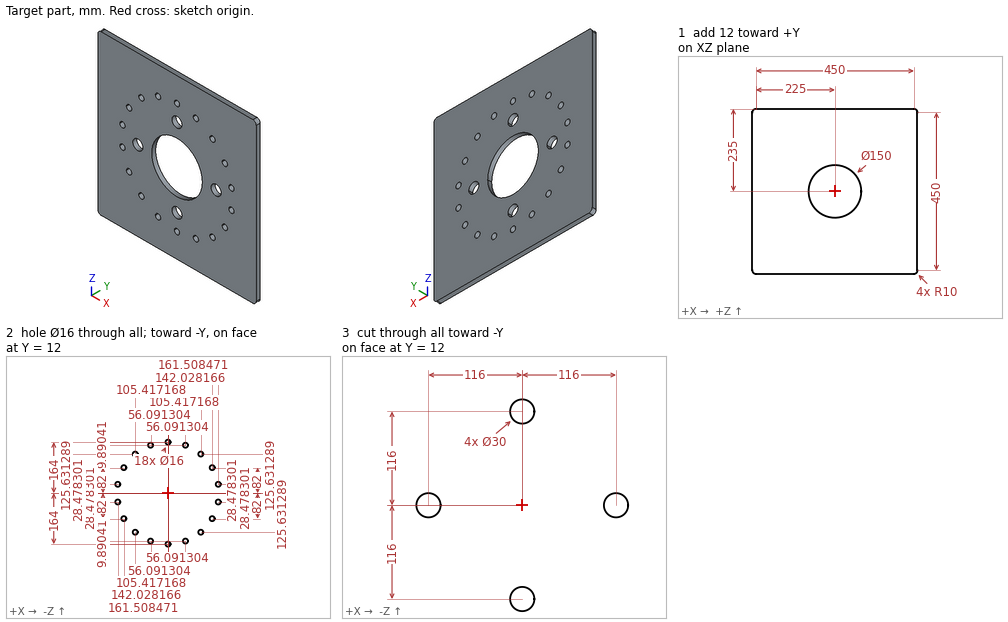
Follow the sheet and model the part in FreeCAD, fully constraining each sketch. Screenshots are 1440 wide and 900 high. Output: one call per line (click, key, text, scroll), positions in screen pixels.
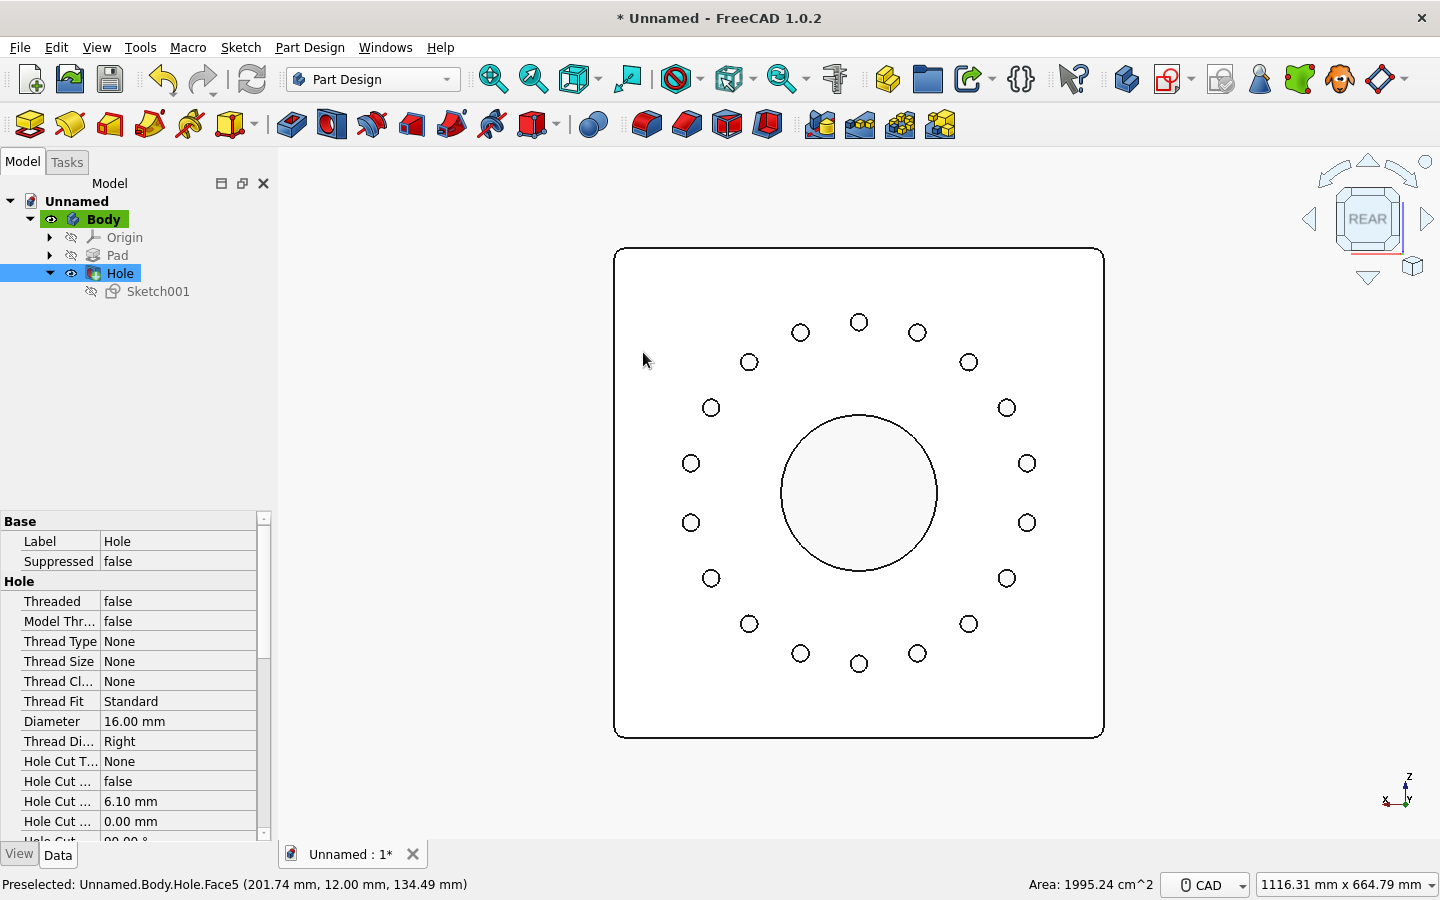
click(1168, 80)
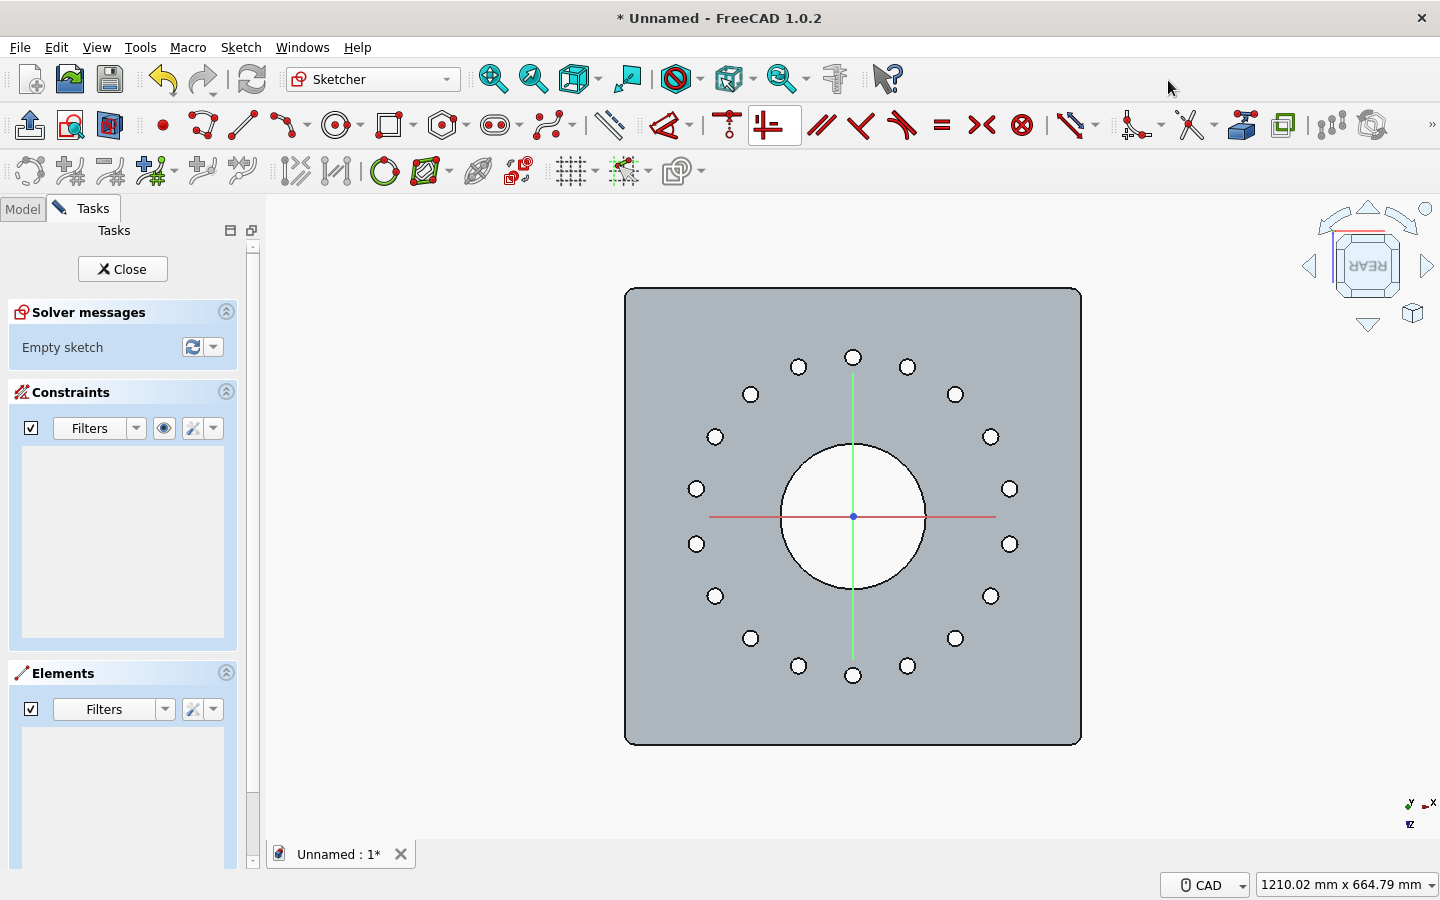
scroll(992, 516, up, 2)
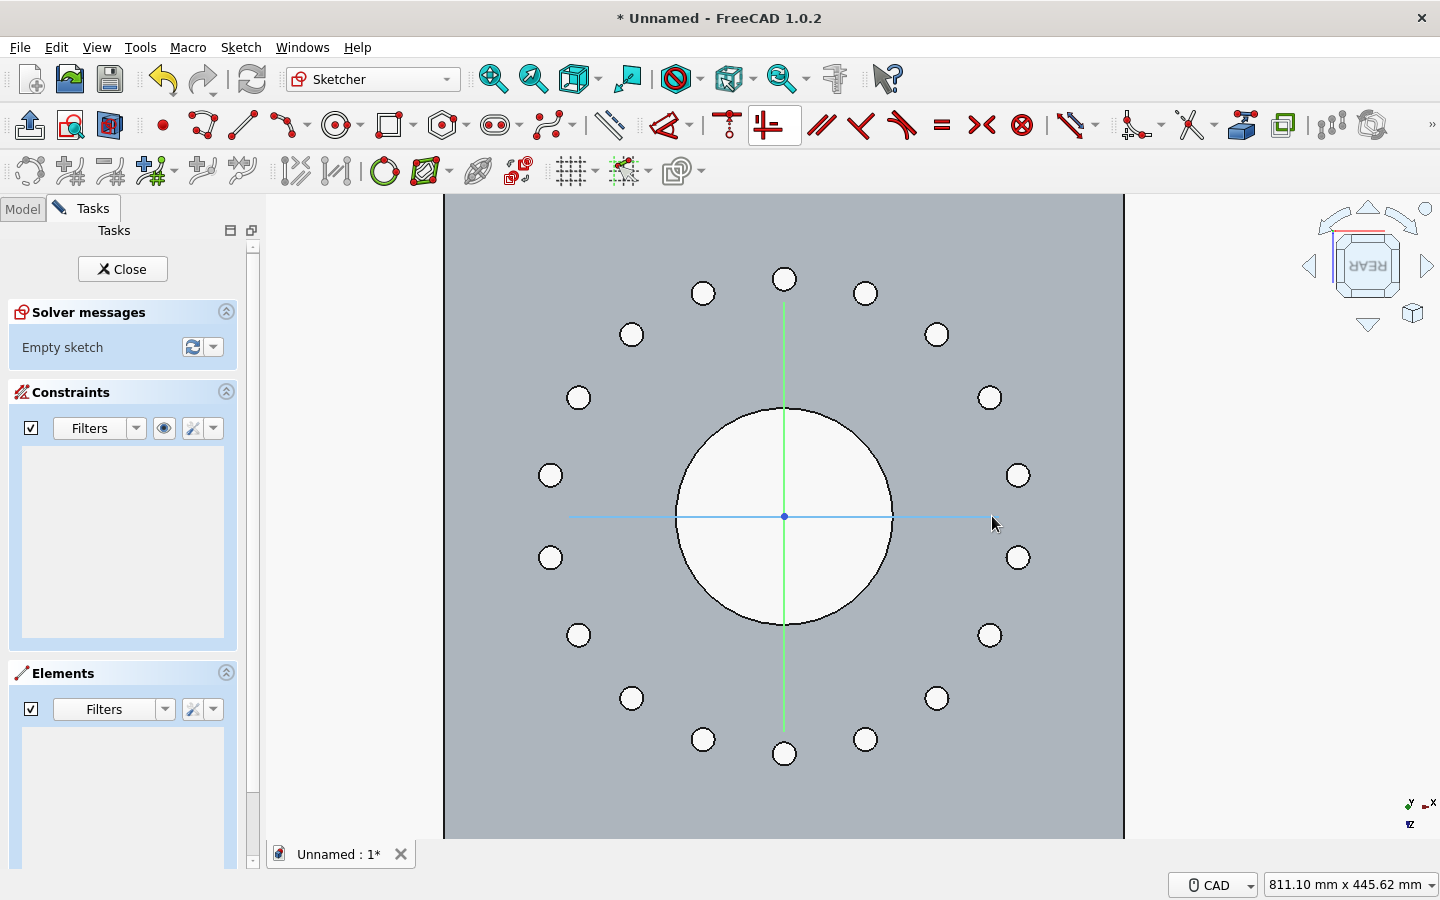
click(336, 126)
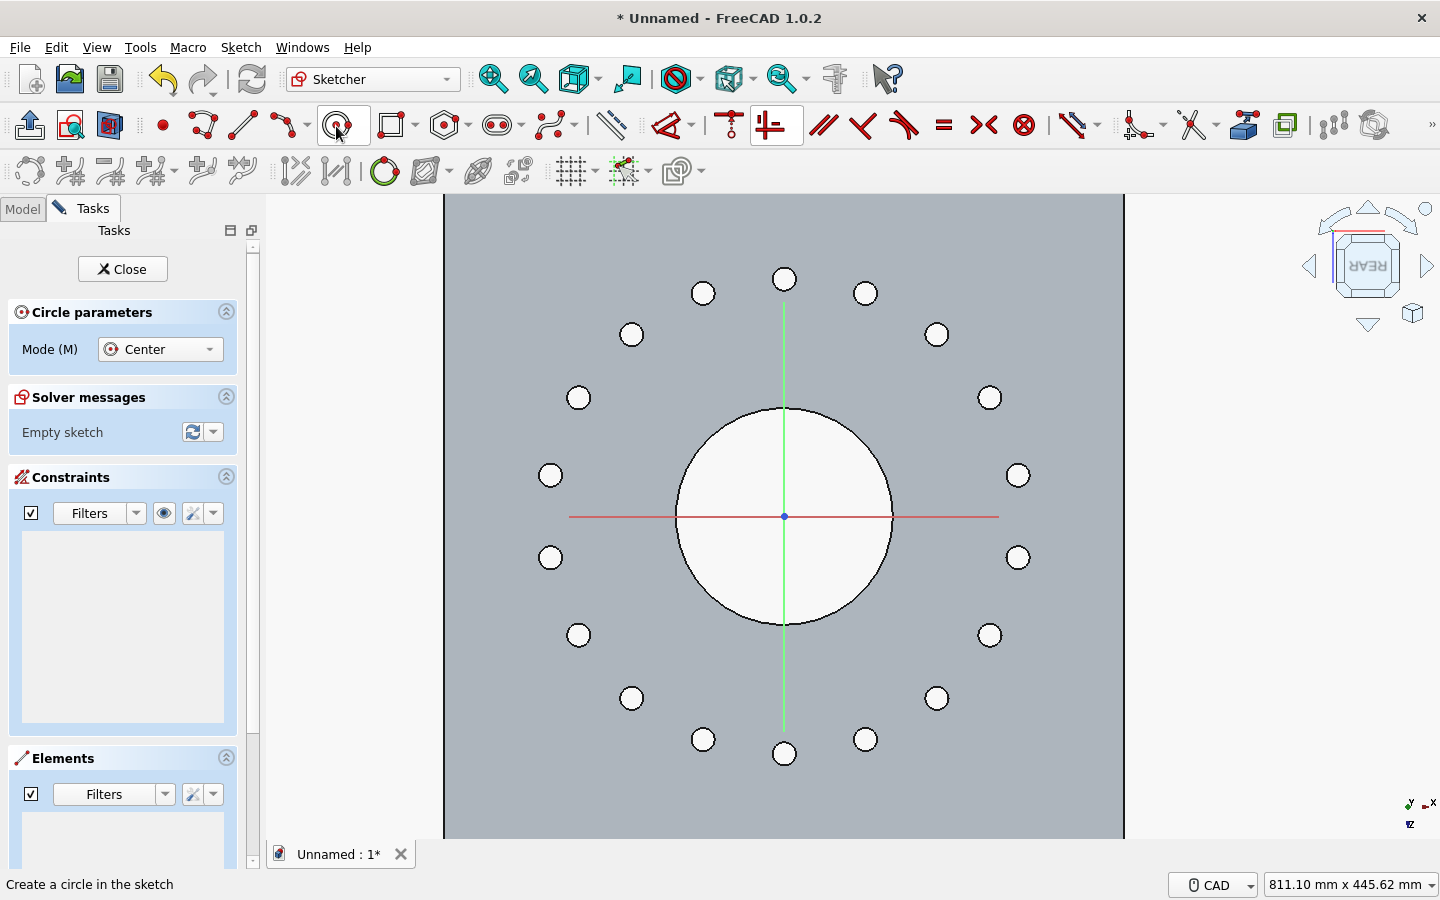
click(784, 349)
move(800, 333)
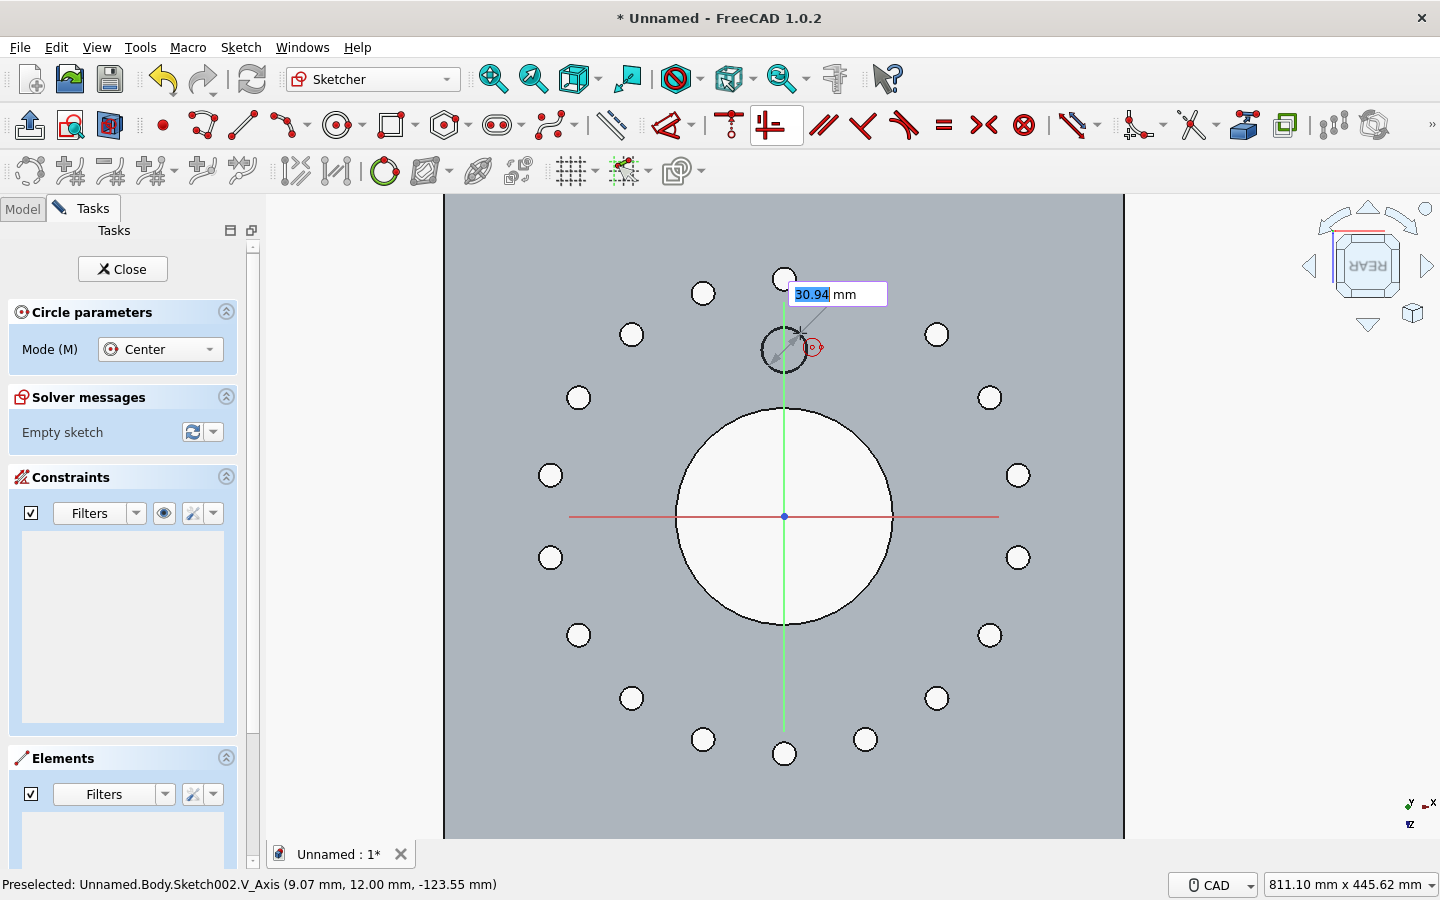
text(30)
key(Return)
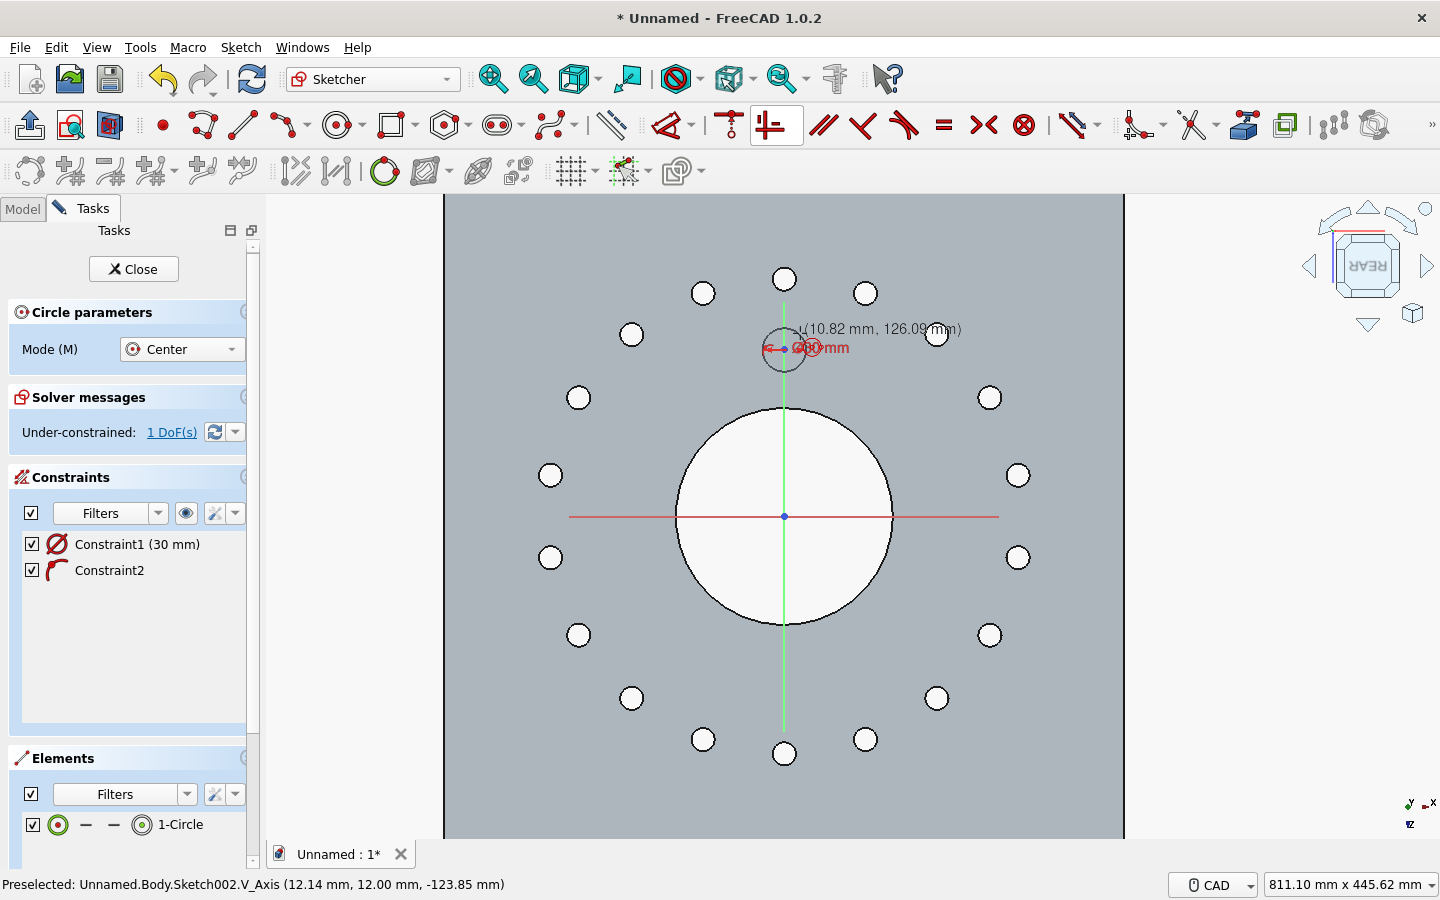
click(952, 516)
move(968, 501)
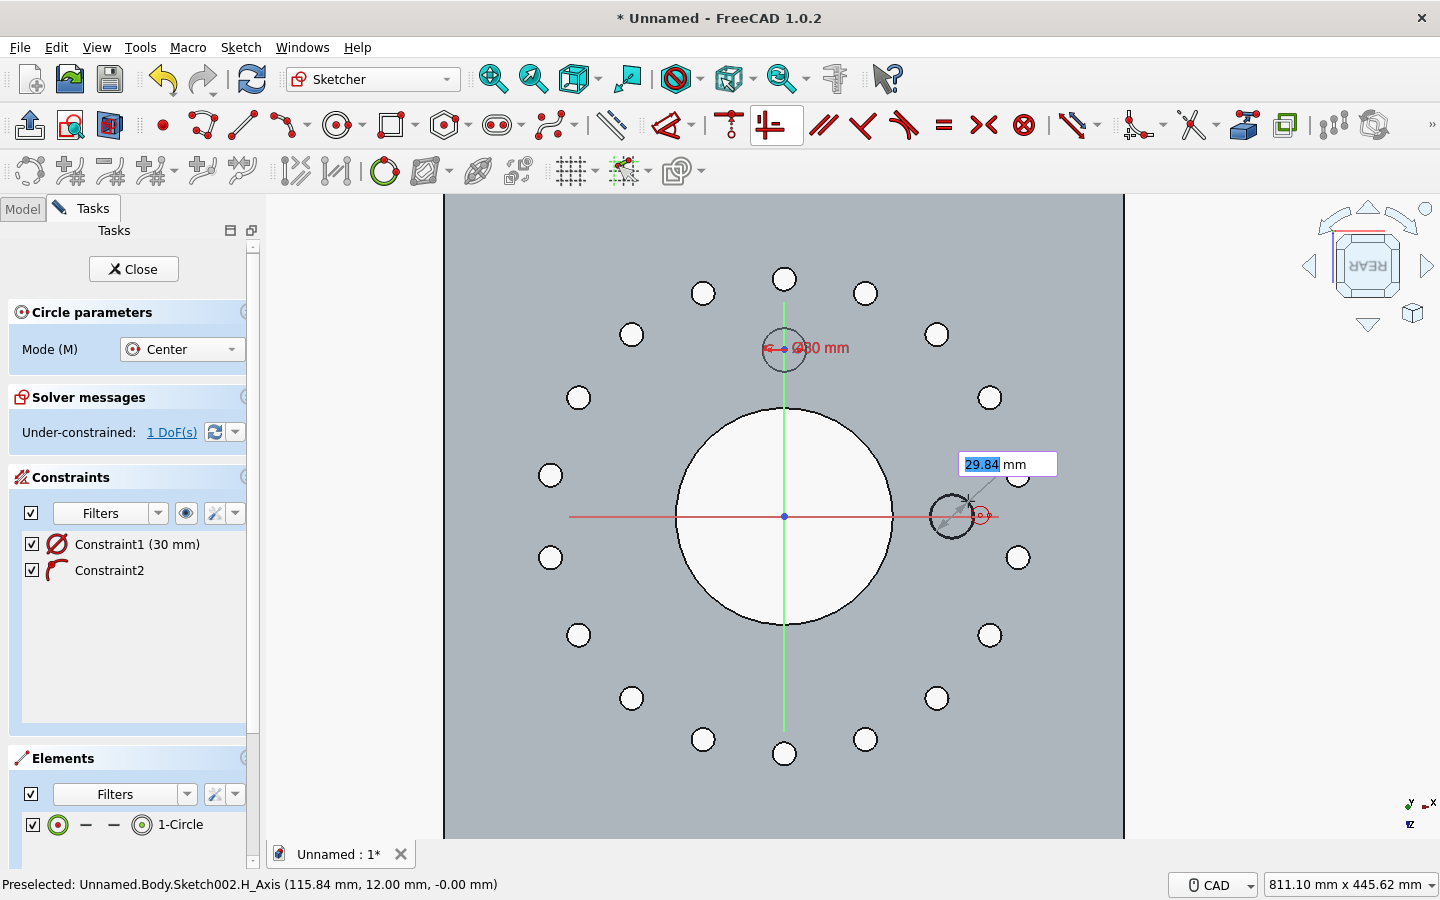
text(30)
key(Return)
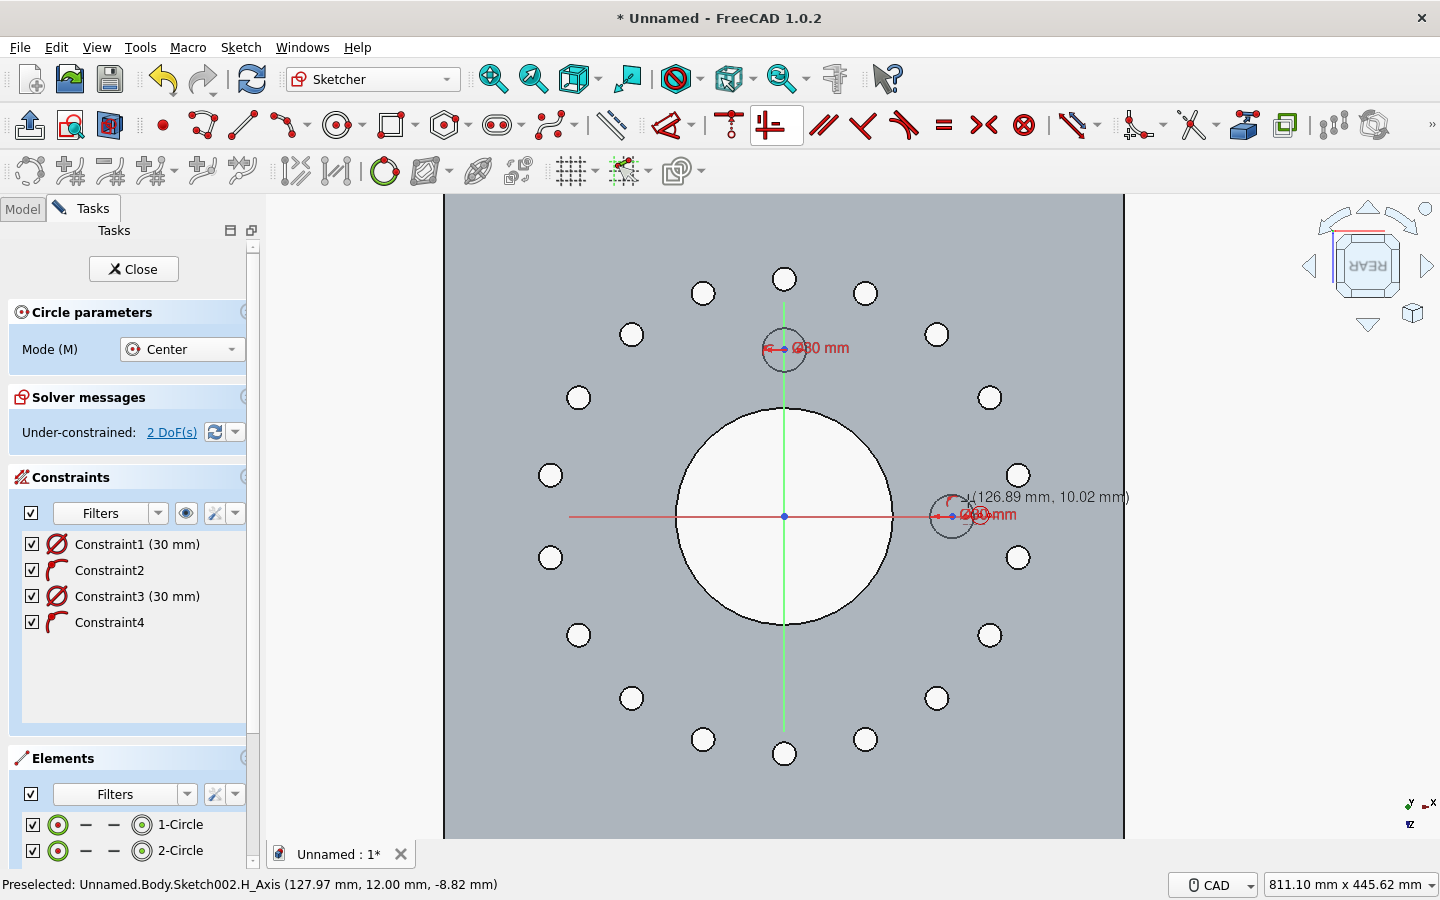
click(784, 684)
move(800, 669)